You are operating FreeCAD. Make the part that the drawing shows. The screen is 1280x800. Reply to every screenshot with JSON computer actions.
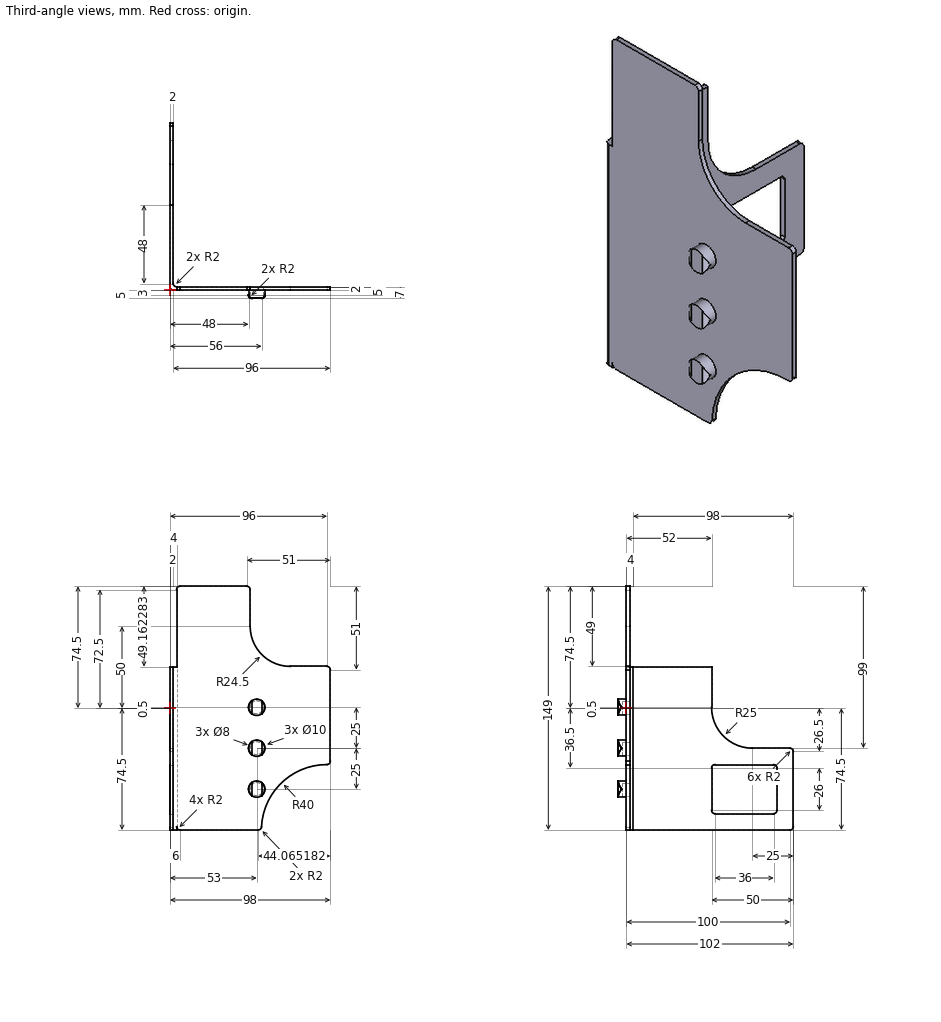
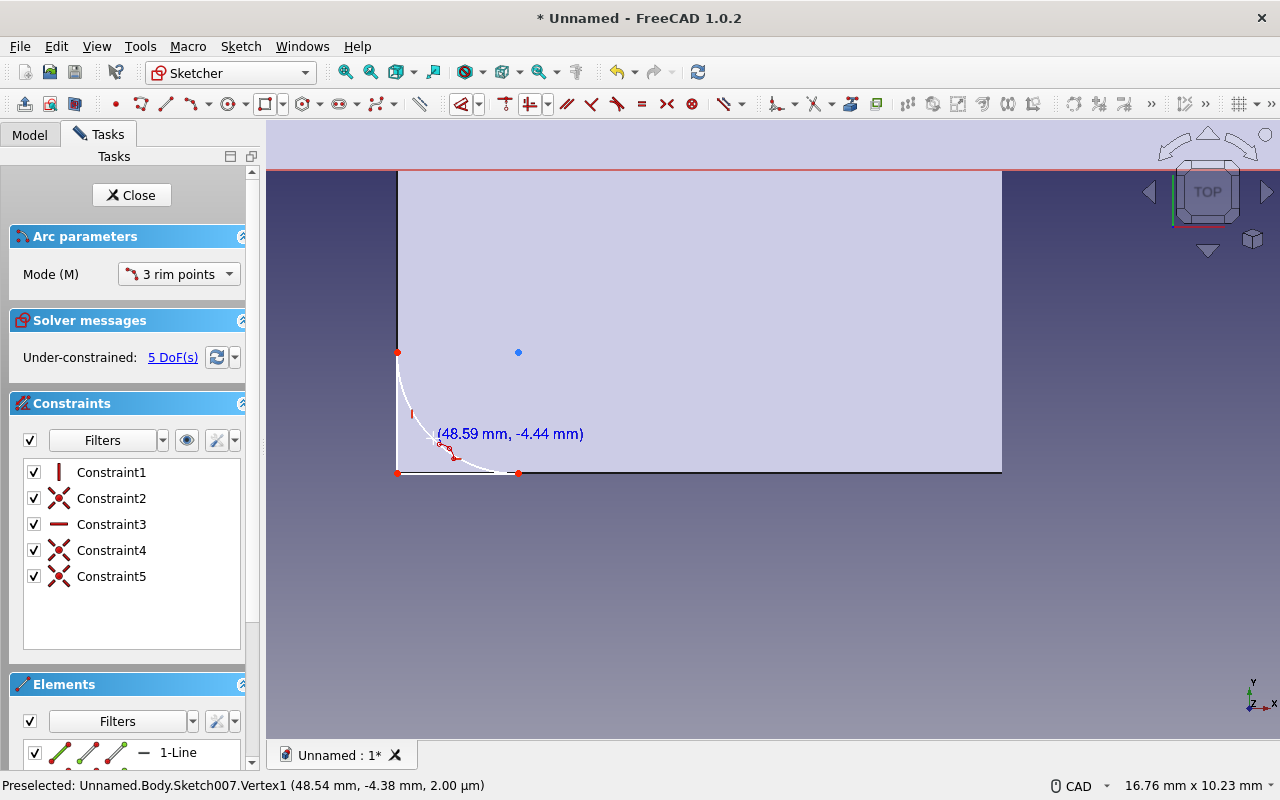
{"action": "key", "text": "g m"}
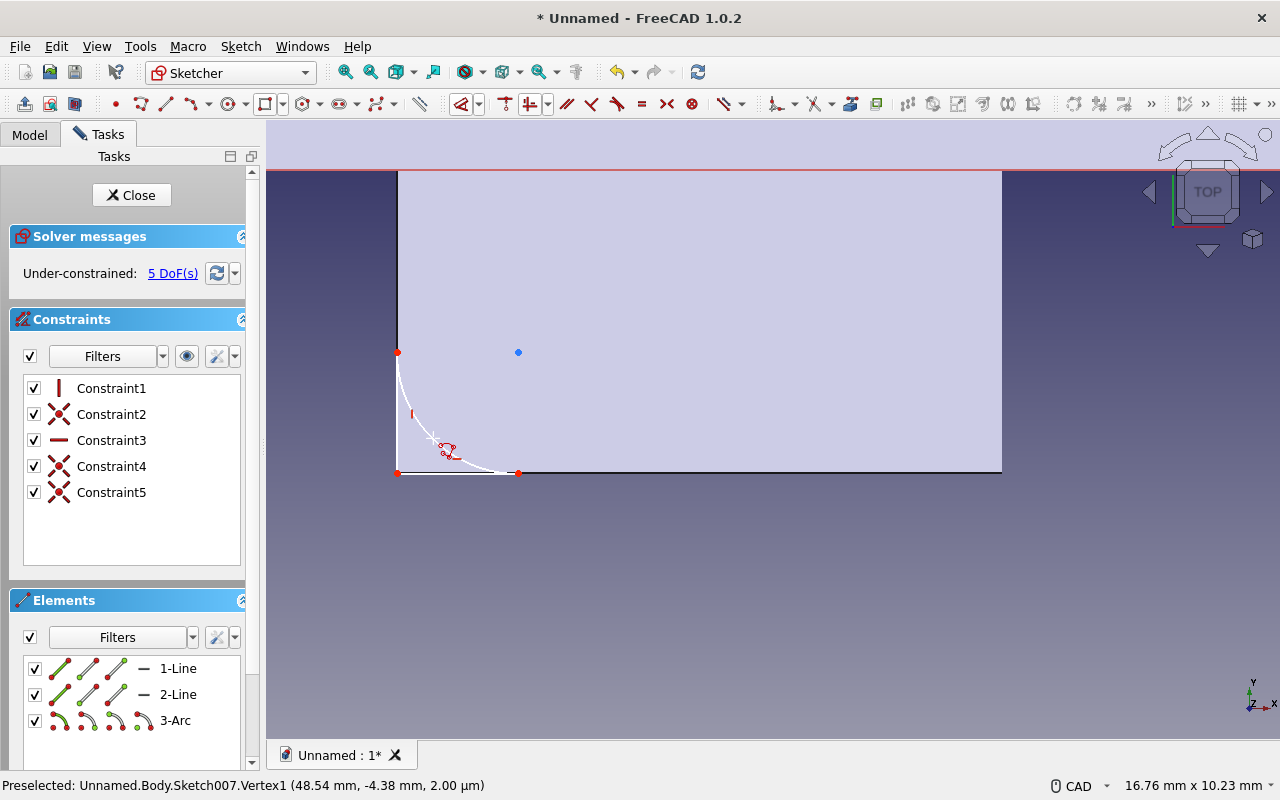
{"action": "left_click", "coordinate": [881, 473]}
{"action": "left_click", "coordinate": [1002, 473]}
{"action": "left_click", "coordinate": [1002, 352]}
{"action": "right_click", "coordinate": [1002, 352]}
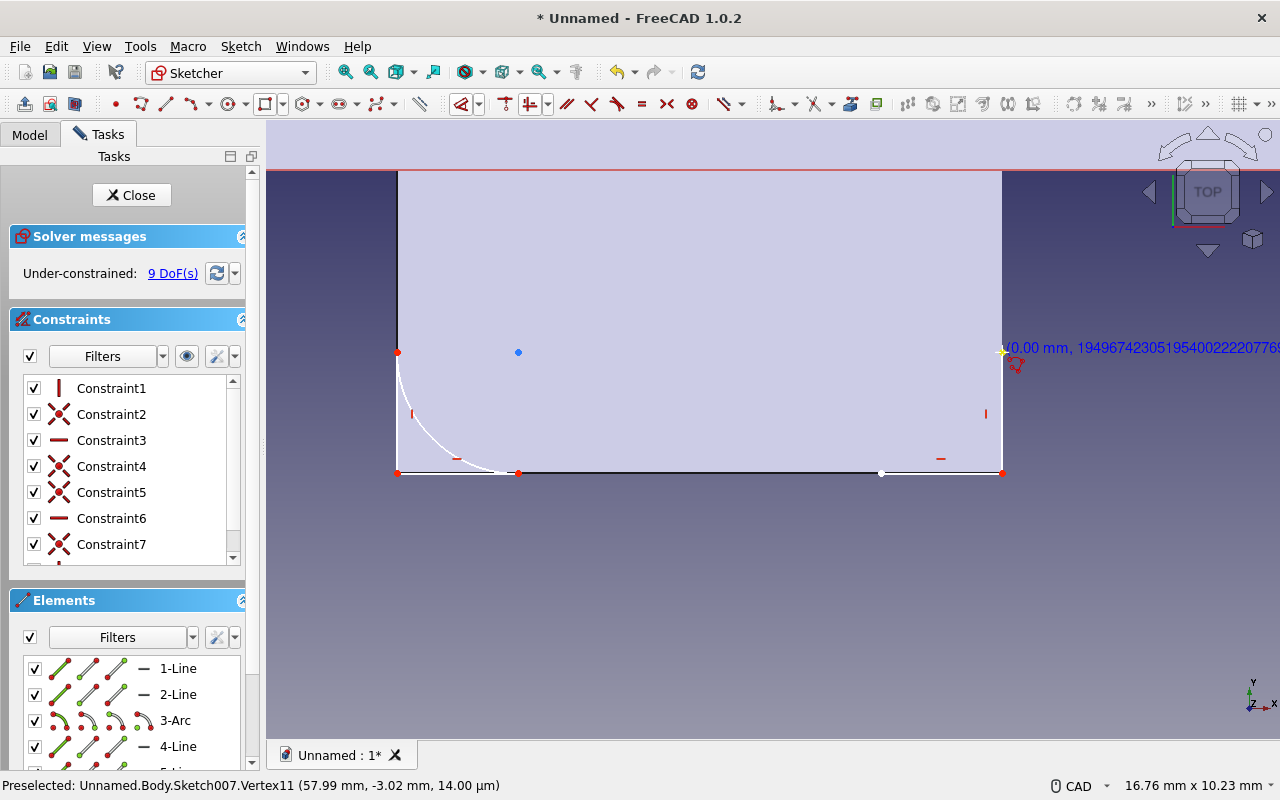
{"action": "left_click", "coordinate": [190, 104]}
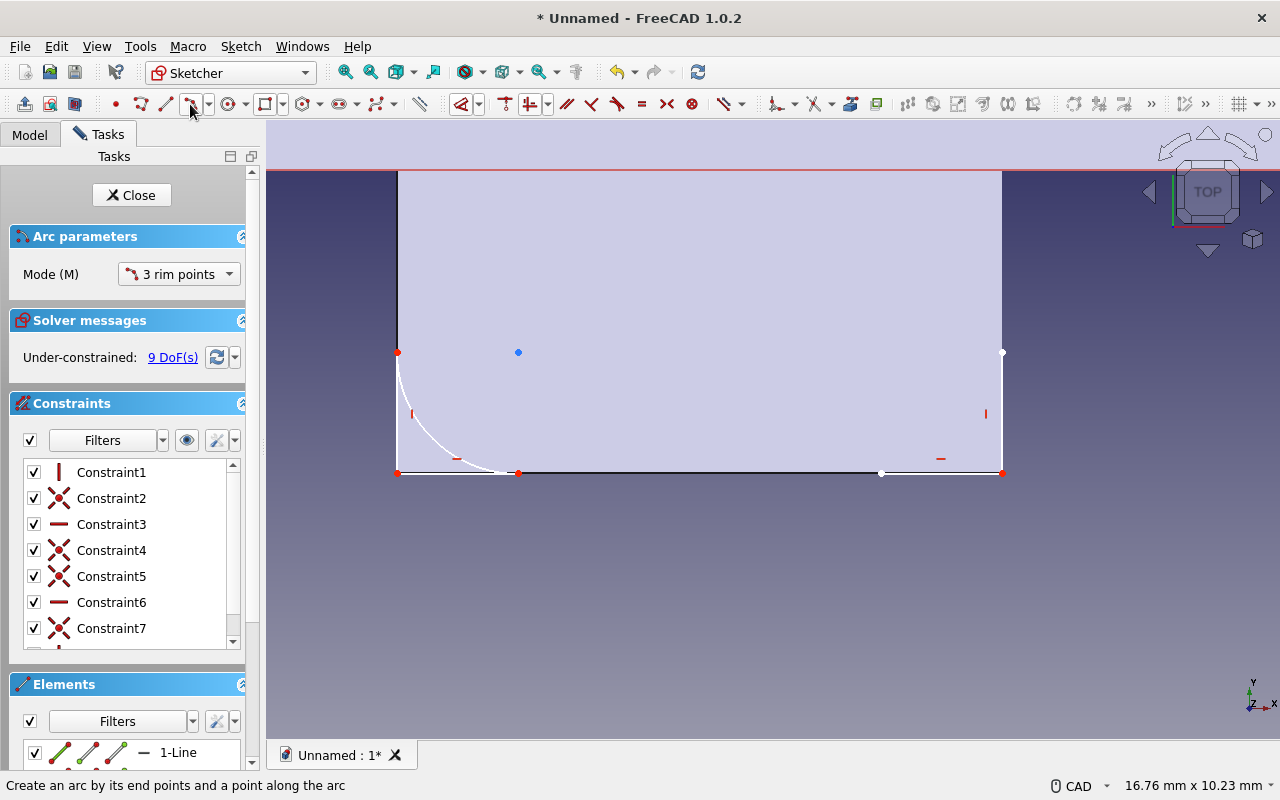
{"action": "left_click", "coordinate": [1002, 353]}
{"action": "left_click", "coordinate": [881, 474]}
{"action": "left_click", "coordinate": [967, 438]}
{"action": "key", "text": "Escape"}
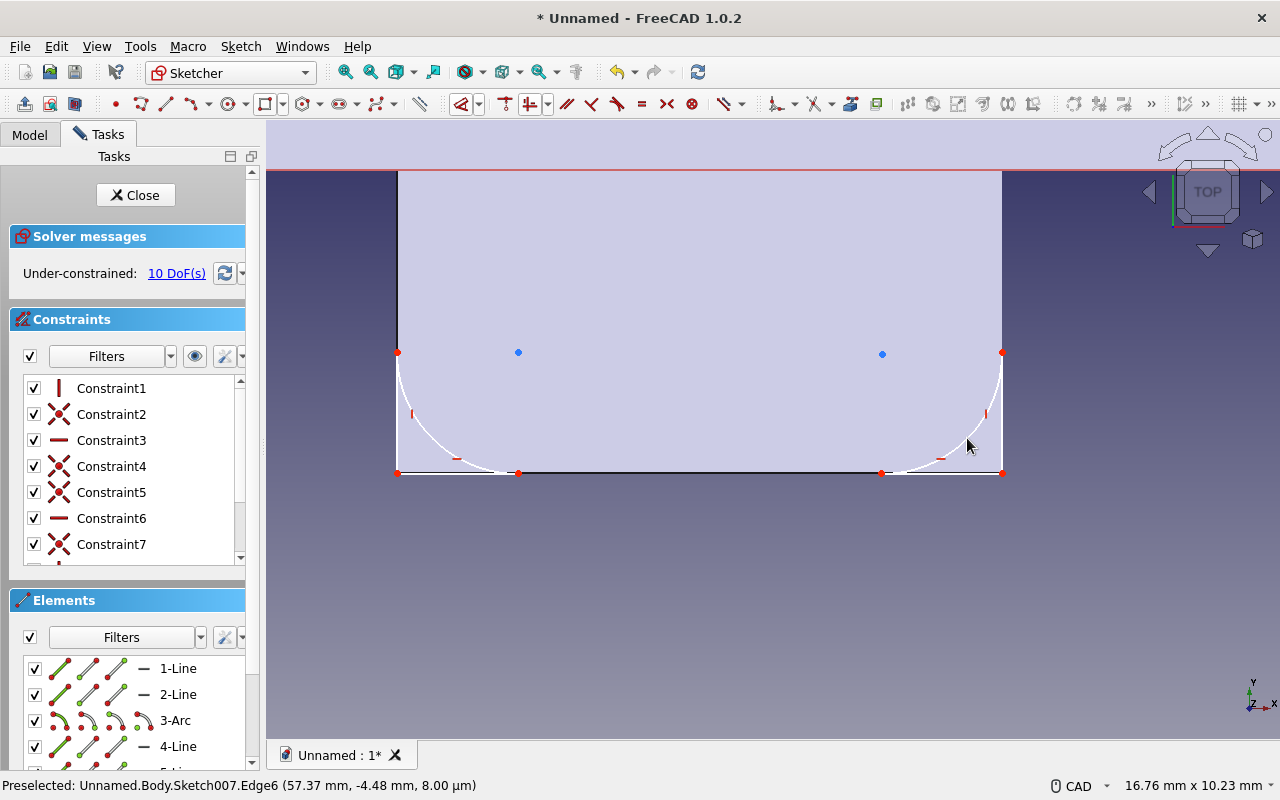
{"action": "left_click", "coordinate": [397, 438]}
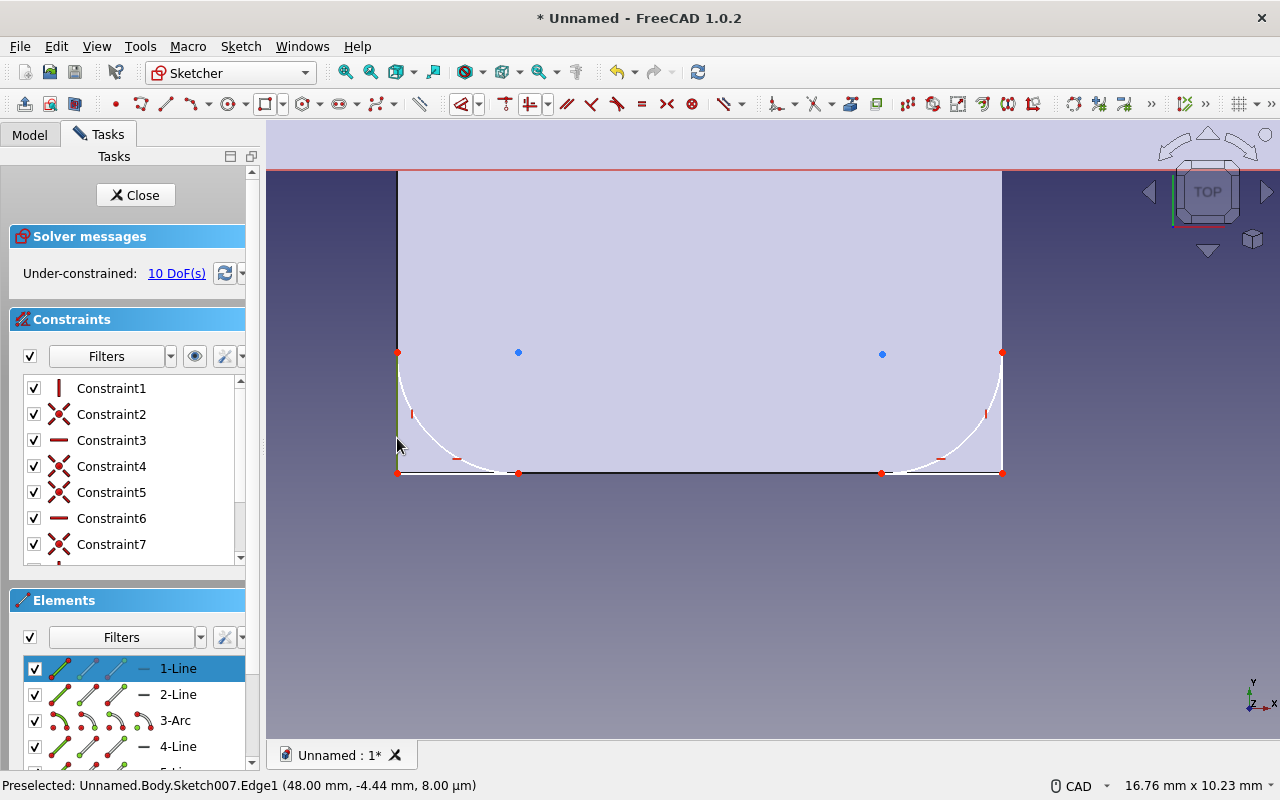
{"action": "left_click", "coordinate": [432, 439]}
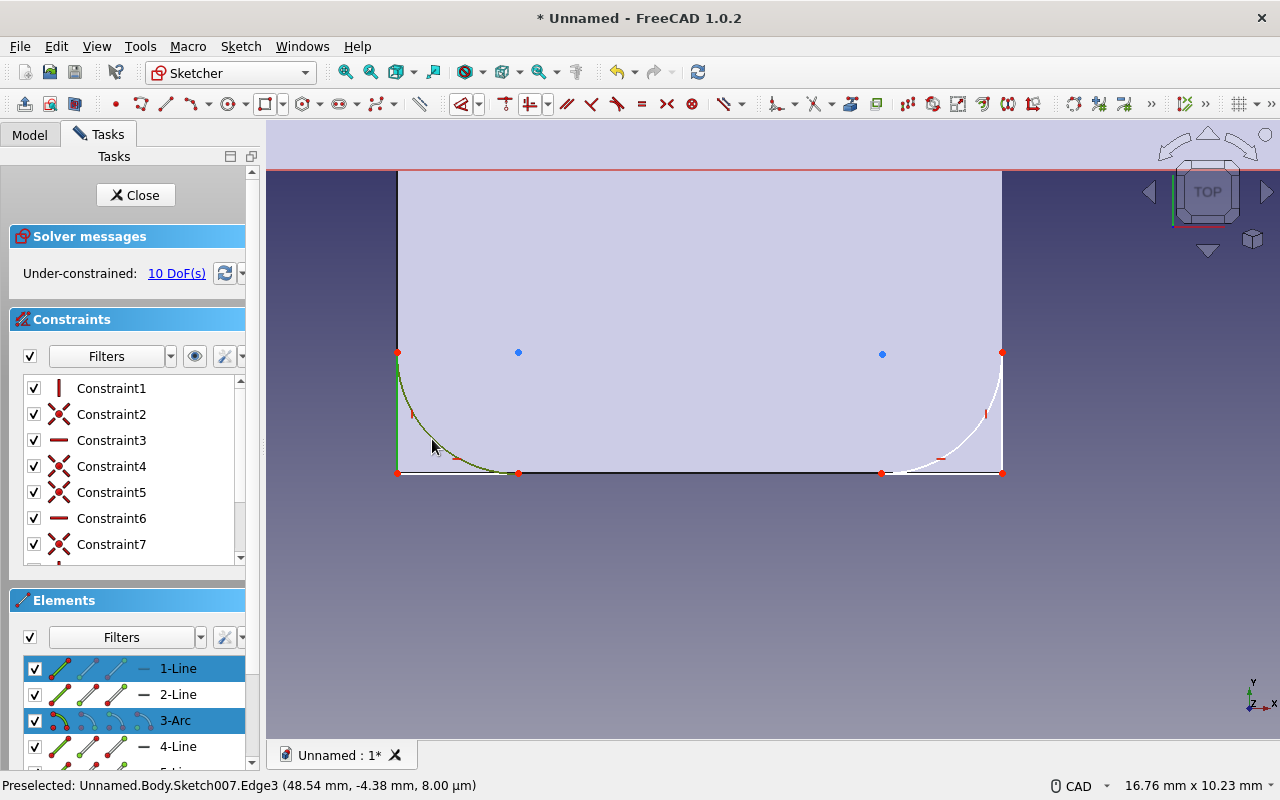
{"action": "key", "text": "t"}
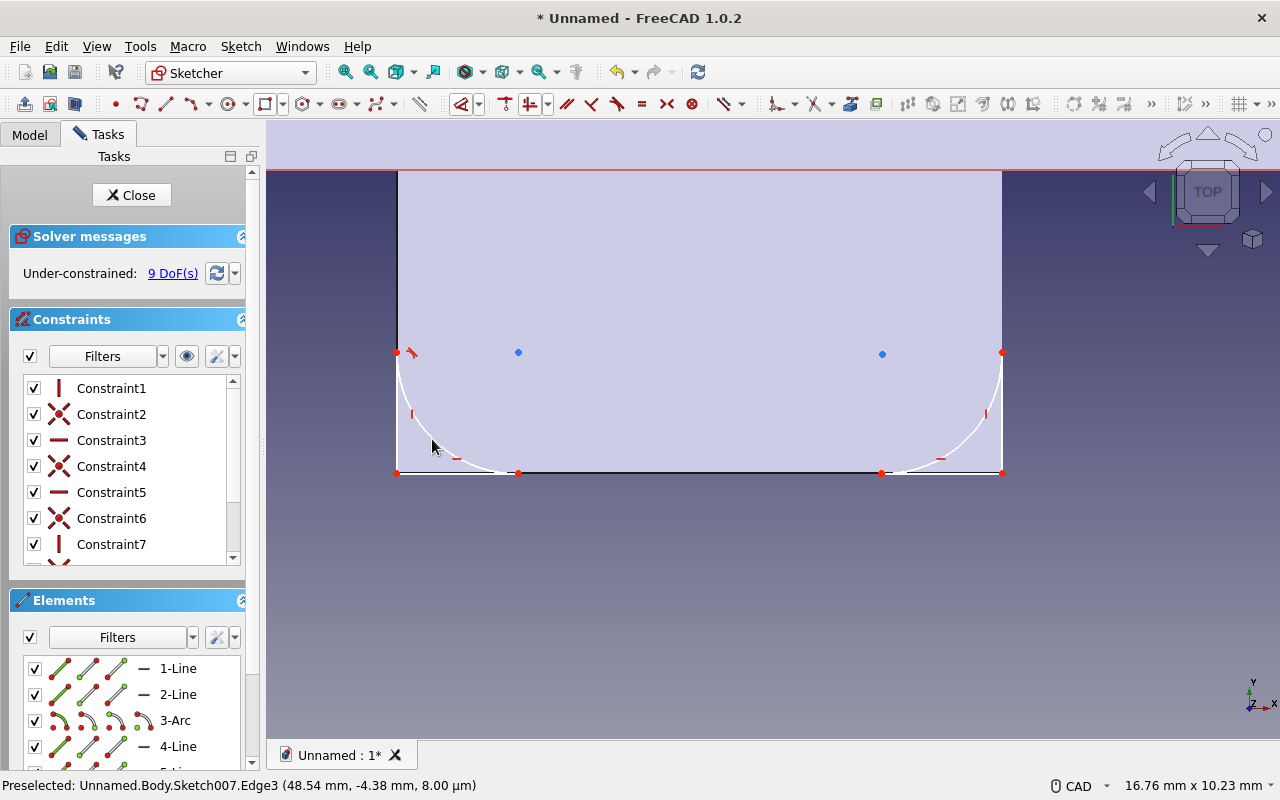
{"action": "left_click", "coordinate": [433, 474]}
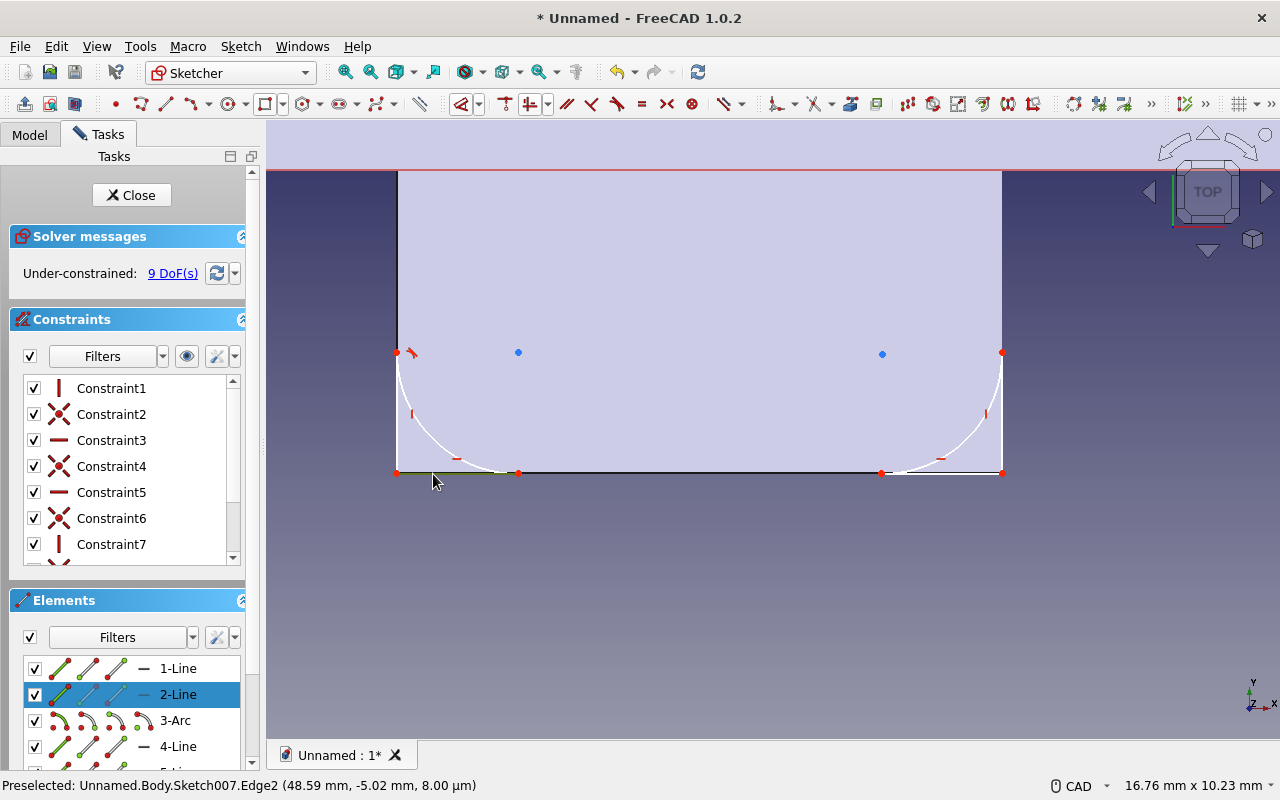
{"action": "left_click", "coordinate": [432, 438]}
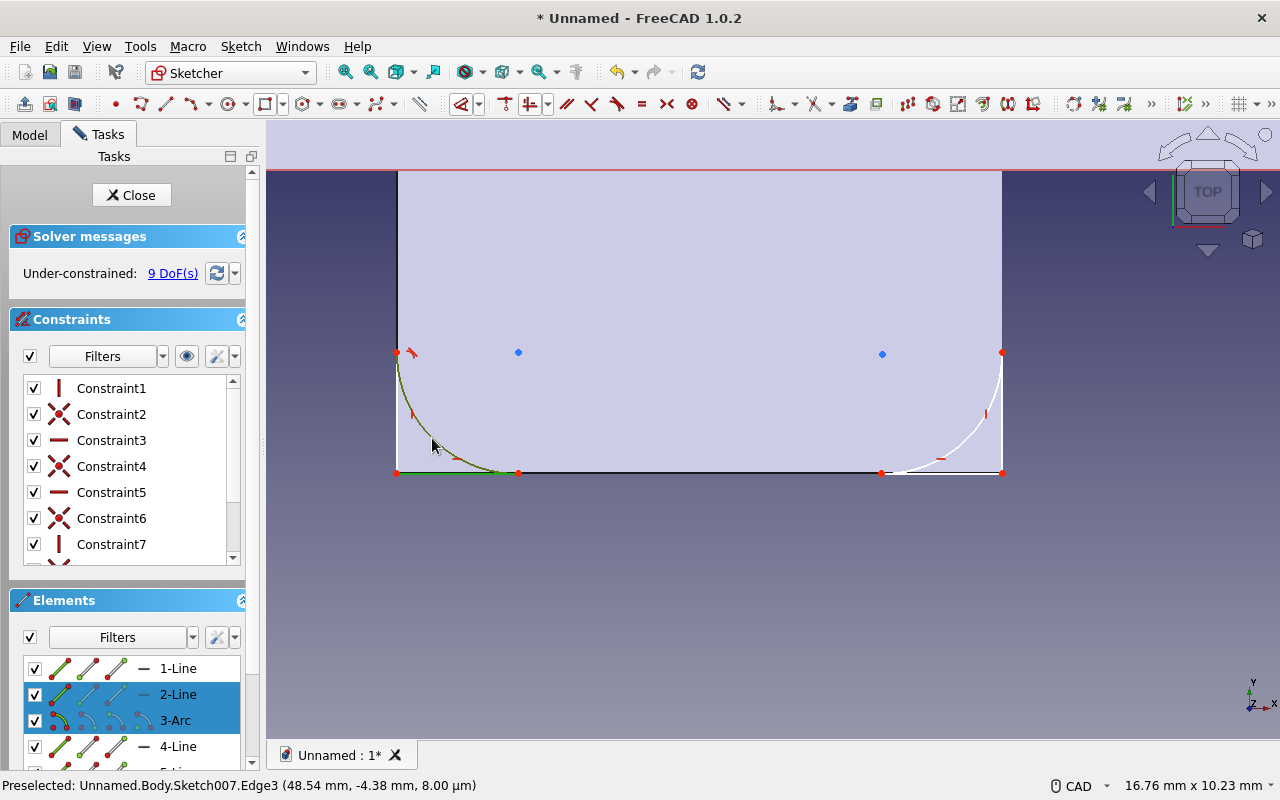
{"action": "key", "text": "t"}